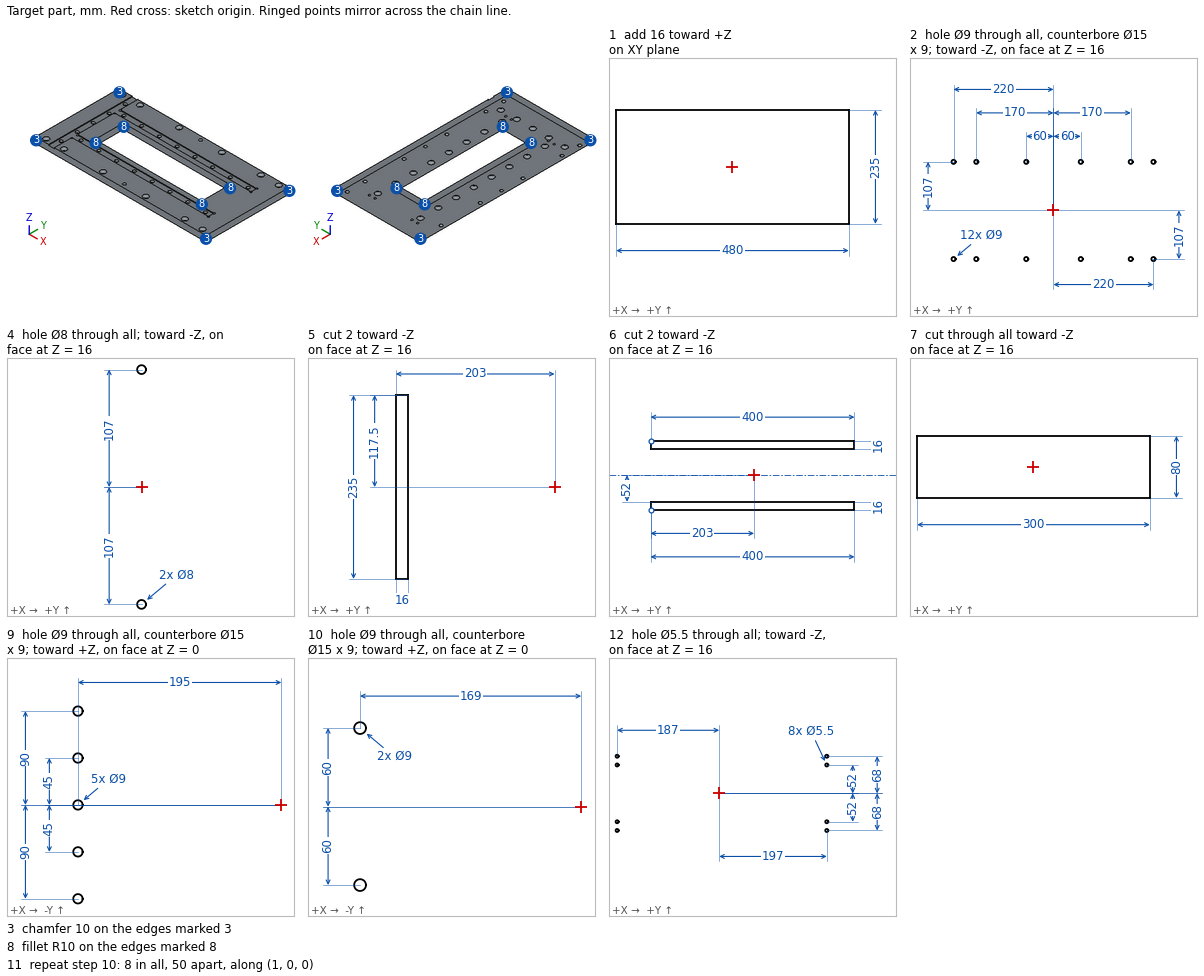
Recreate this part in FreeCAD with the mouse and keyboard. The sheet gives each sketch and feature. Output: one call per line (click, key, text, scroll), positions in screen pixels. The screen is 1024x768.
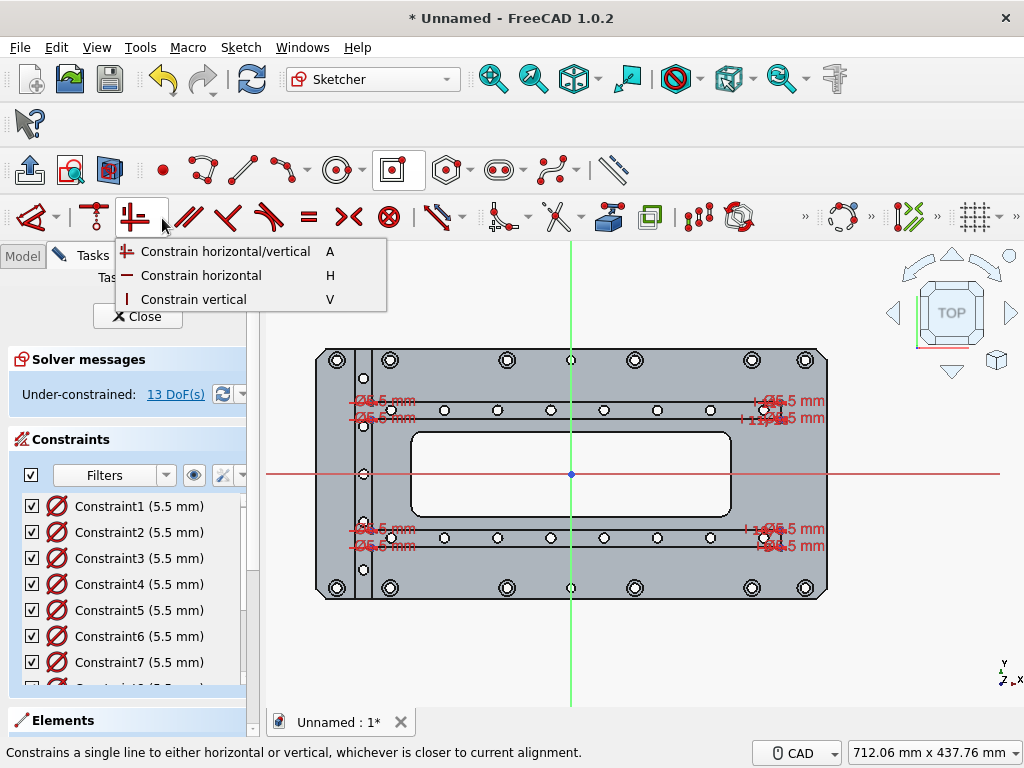
click(251, 275)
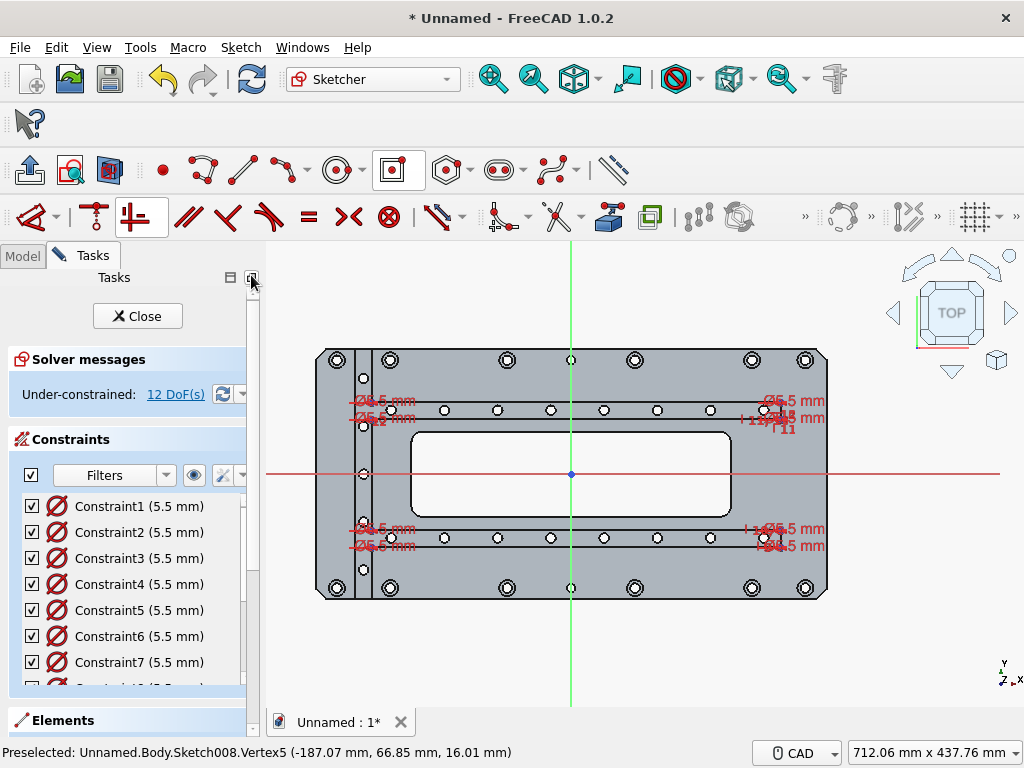
click(372, 403)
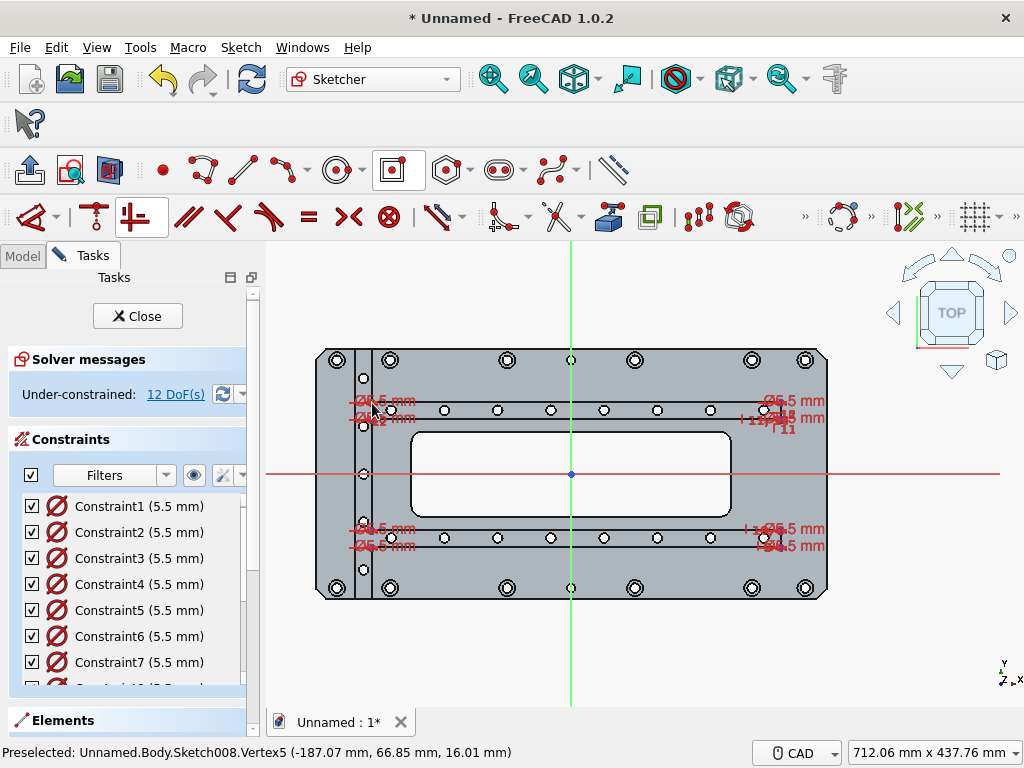
scroll(372, 420, up, 4)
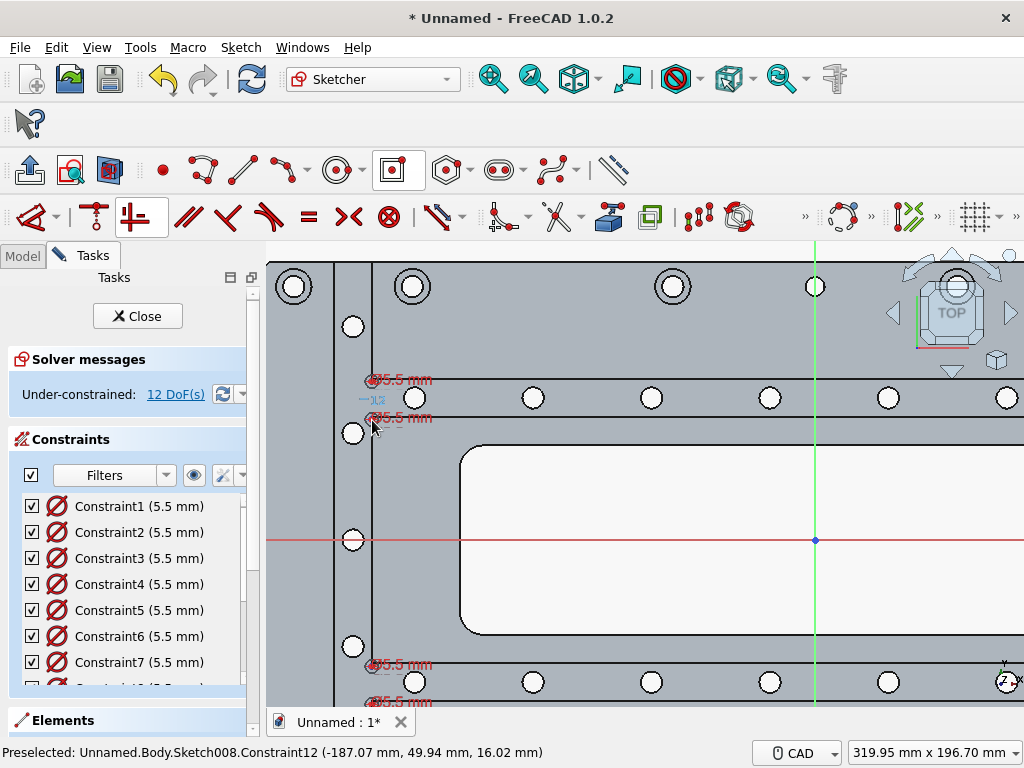
click(372, 420)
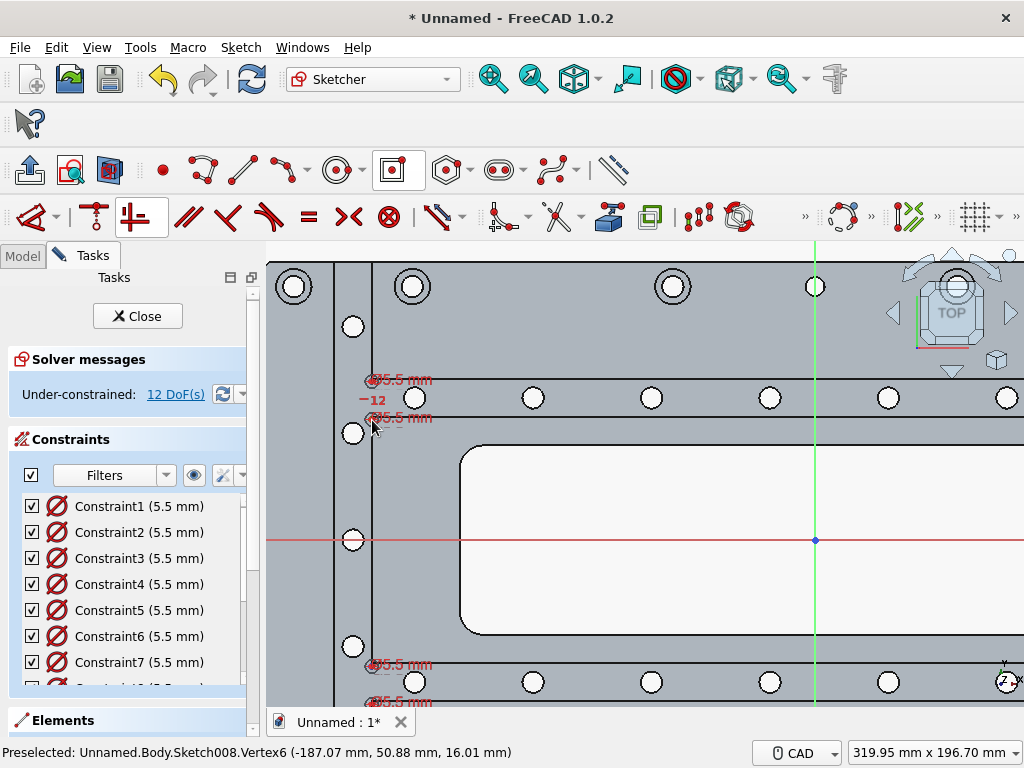
key(v)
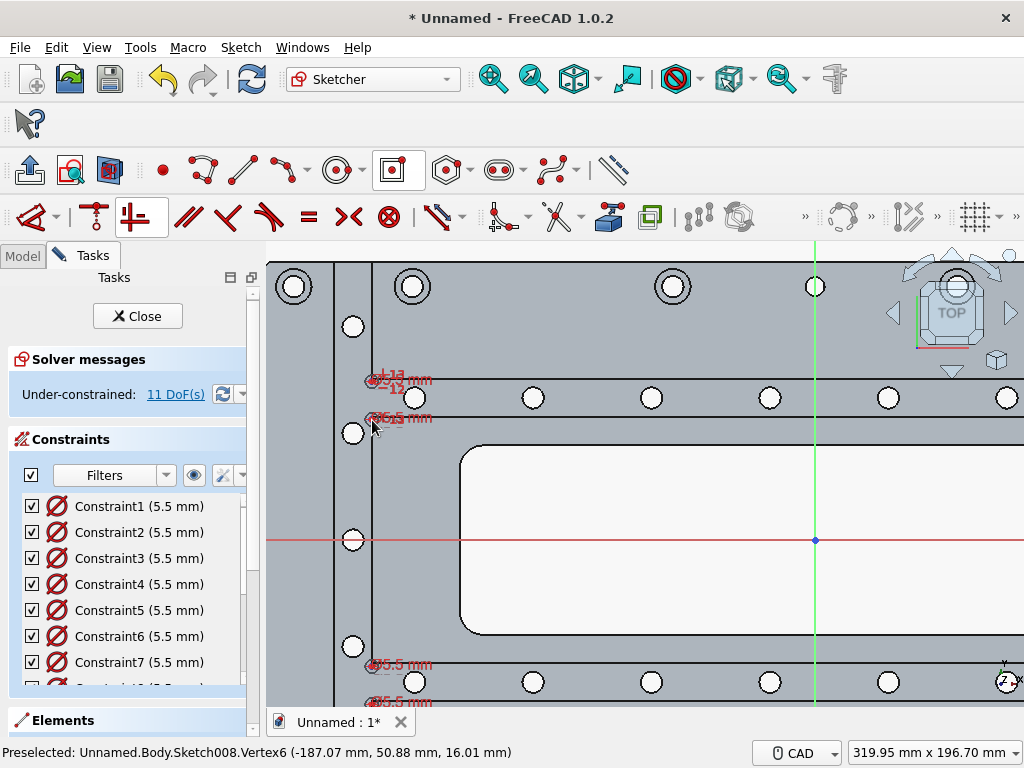
scroll(372, 420, down, 4)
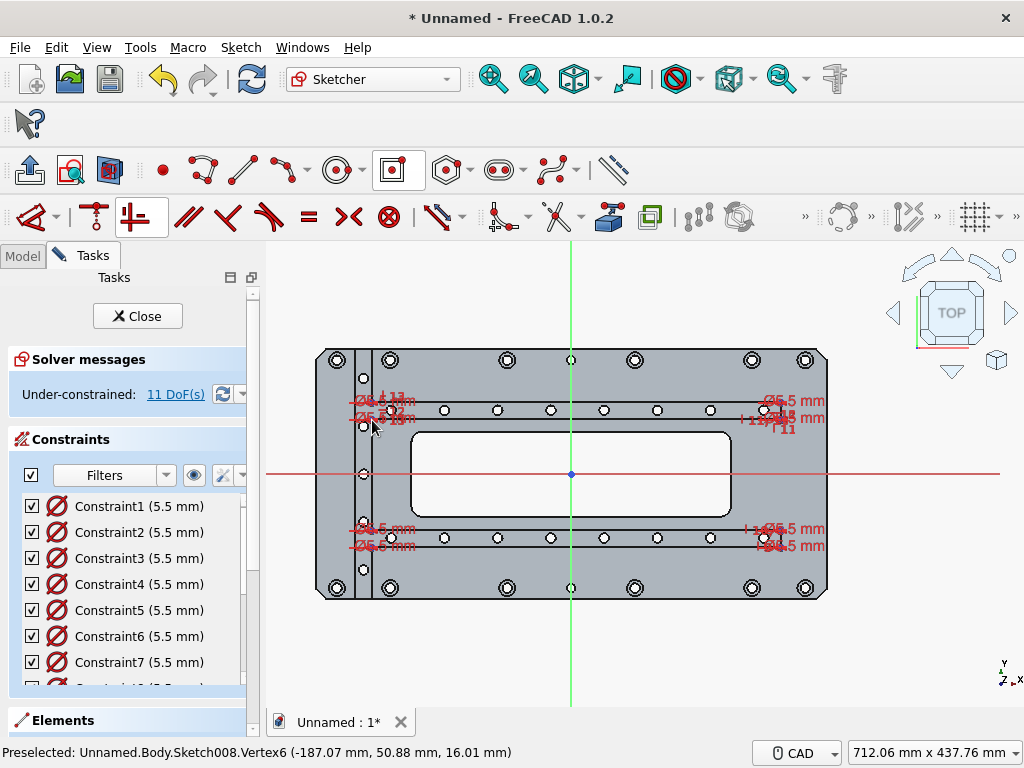
click(781, 420)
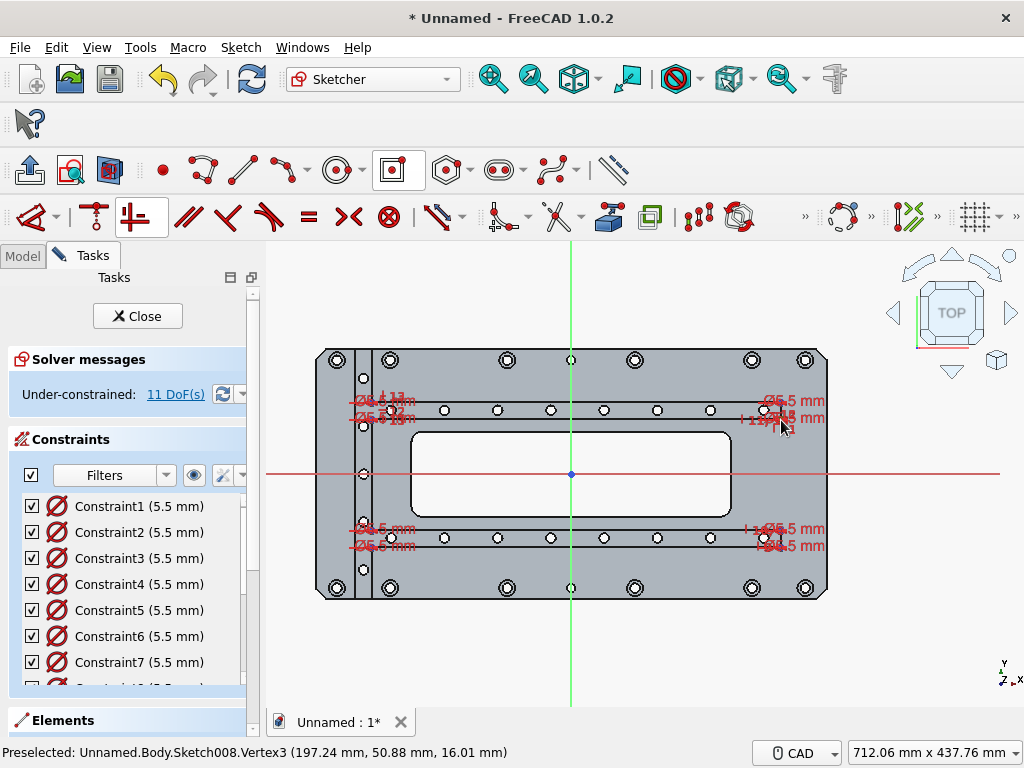
click(372, 420)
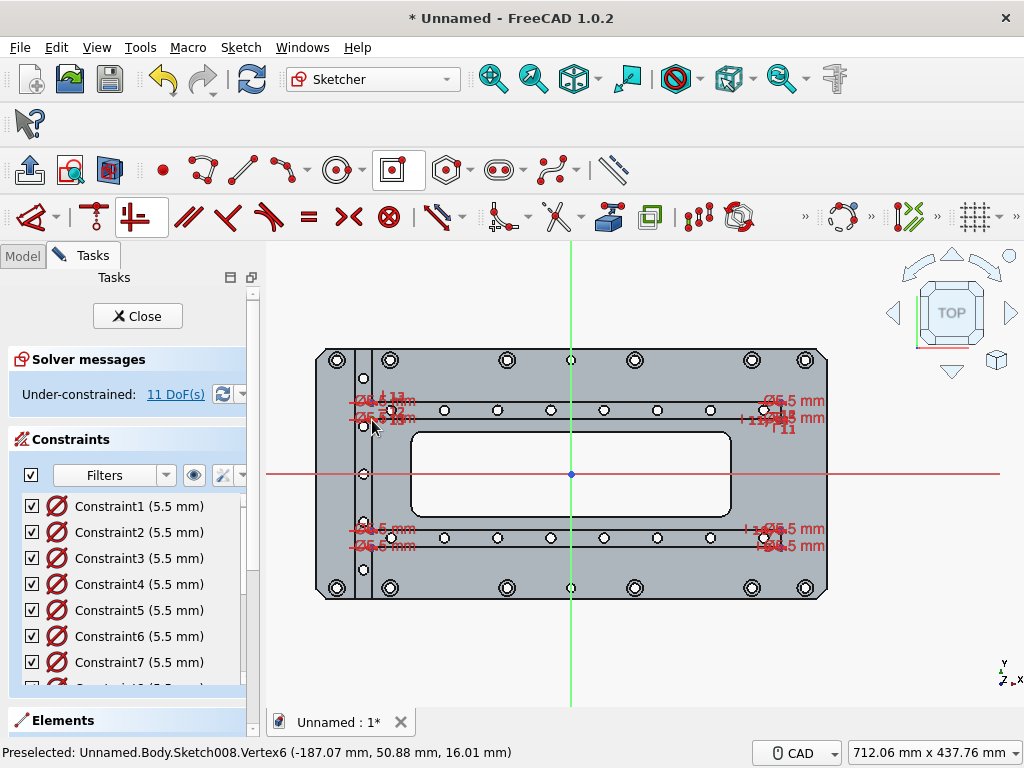
click(162, 218)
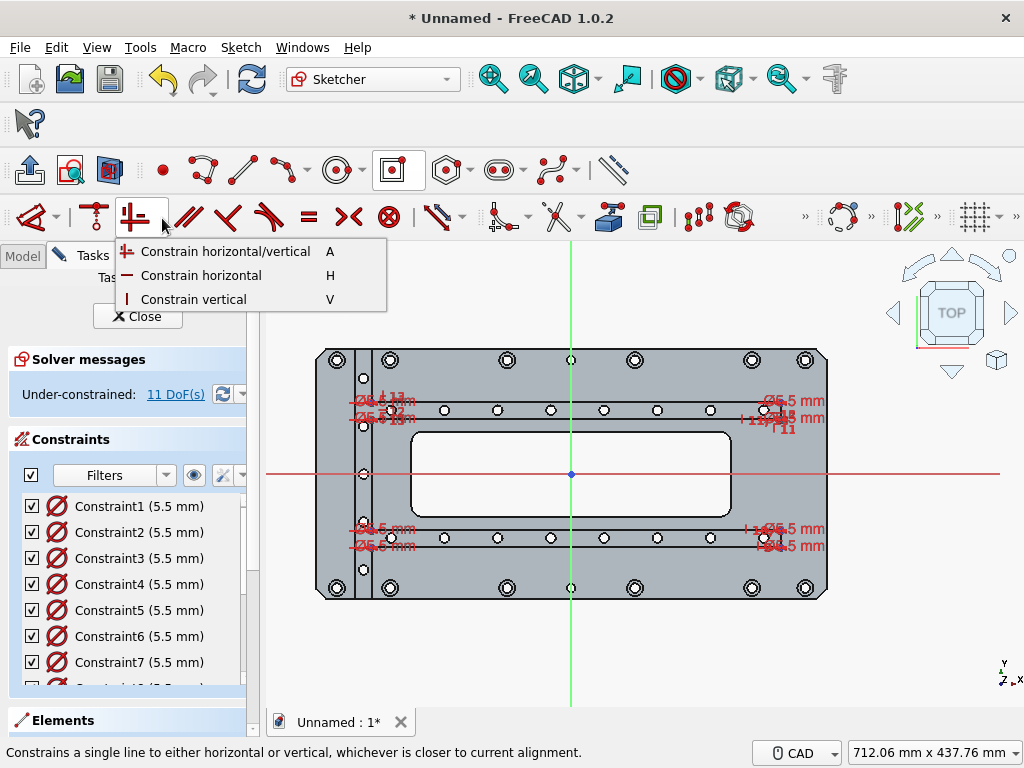
click(251, 275)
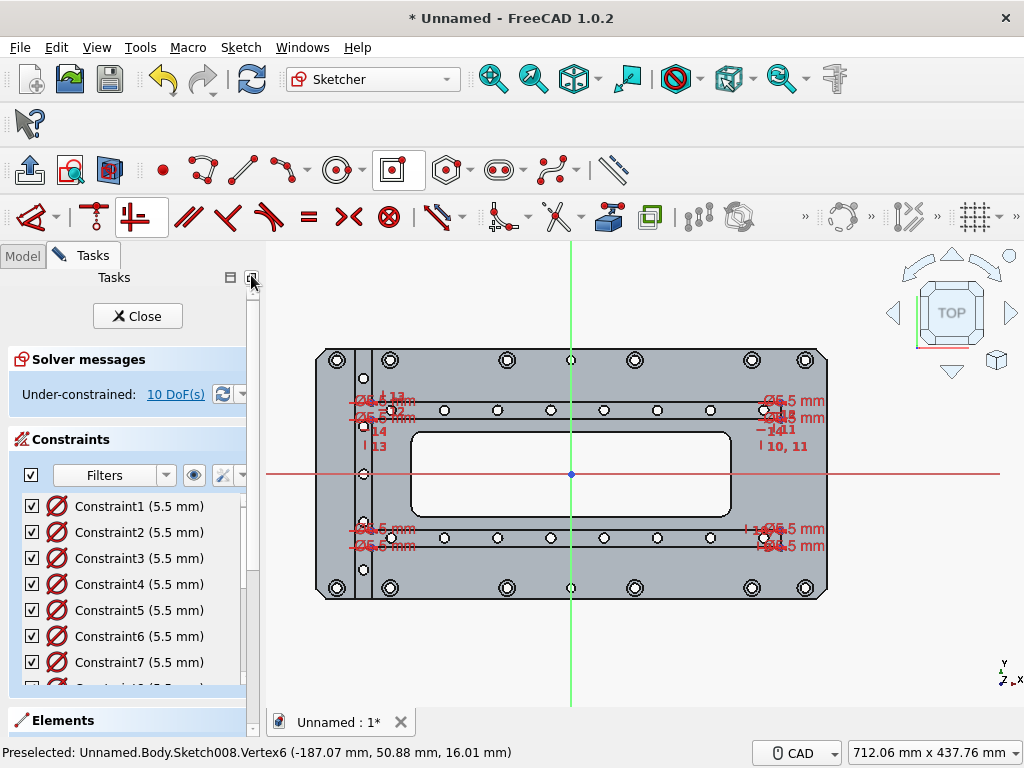
click(372, 420)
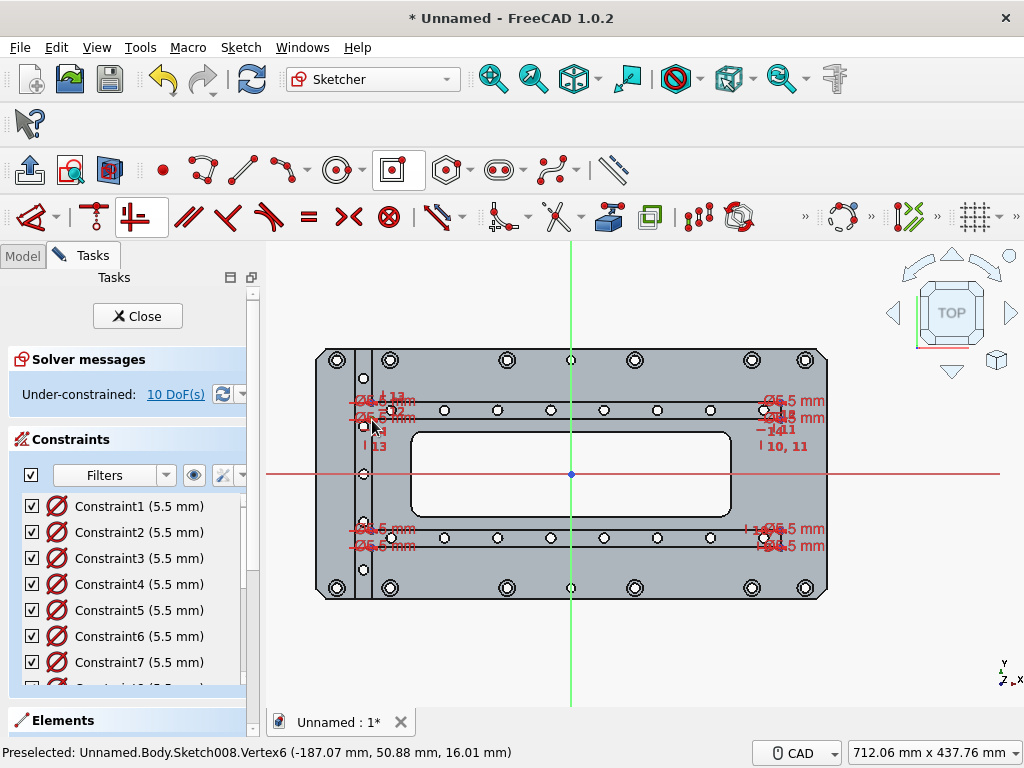
click(372, 548)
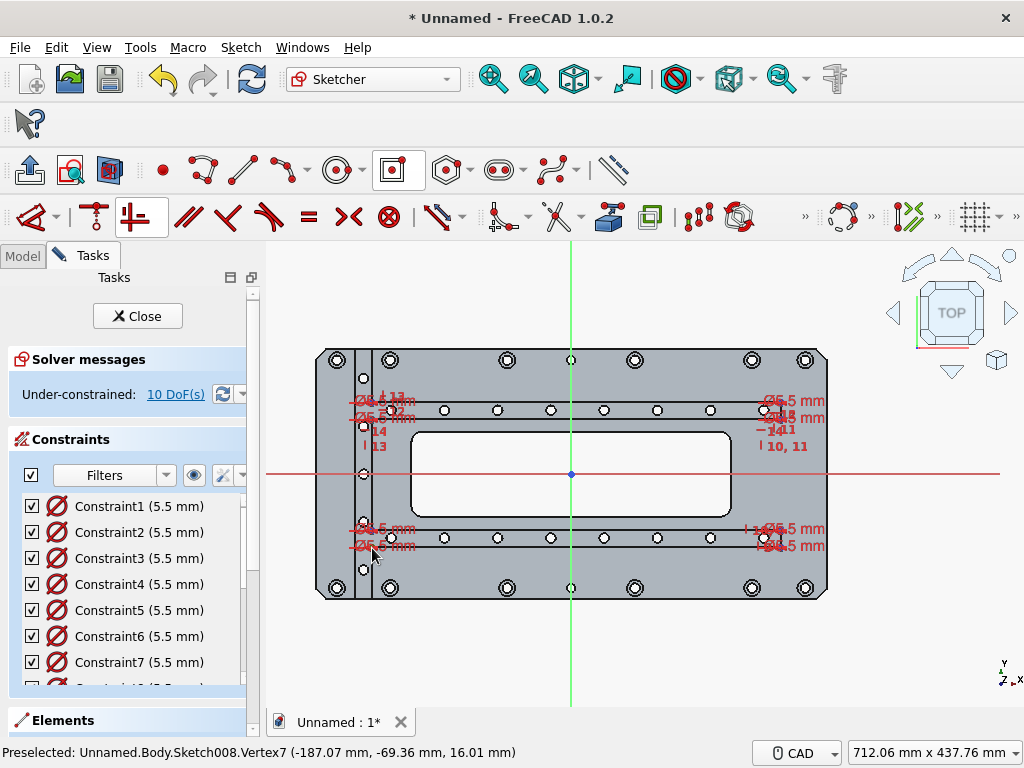
key(v)